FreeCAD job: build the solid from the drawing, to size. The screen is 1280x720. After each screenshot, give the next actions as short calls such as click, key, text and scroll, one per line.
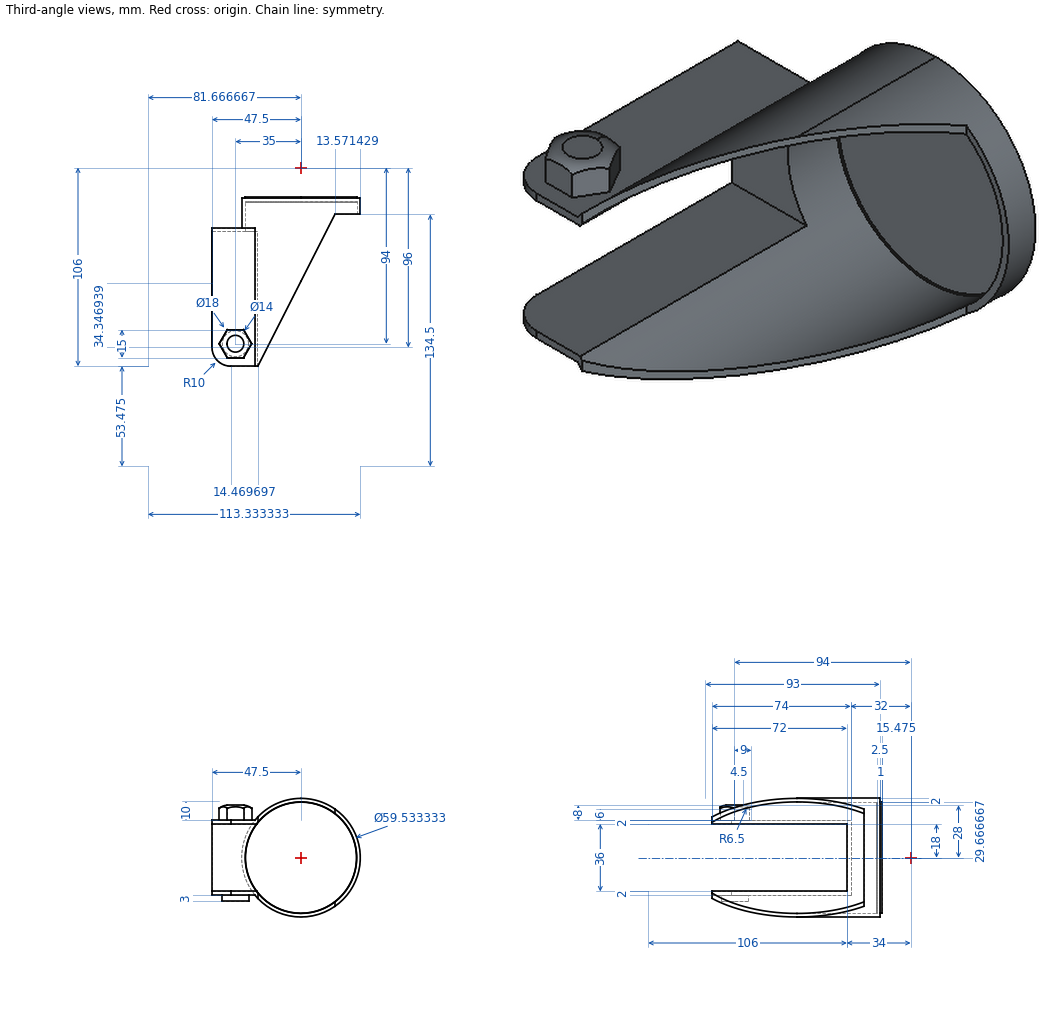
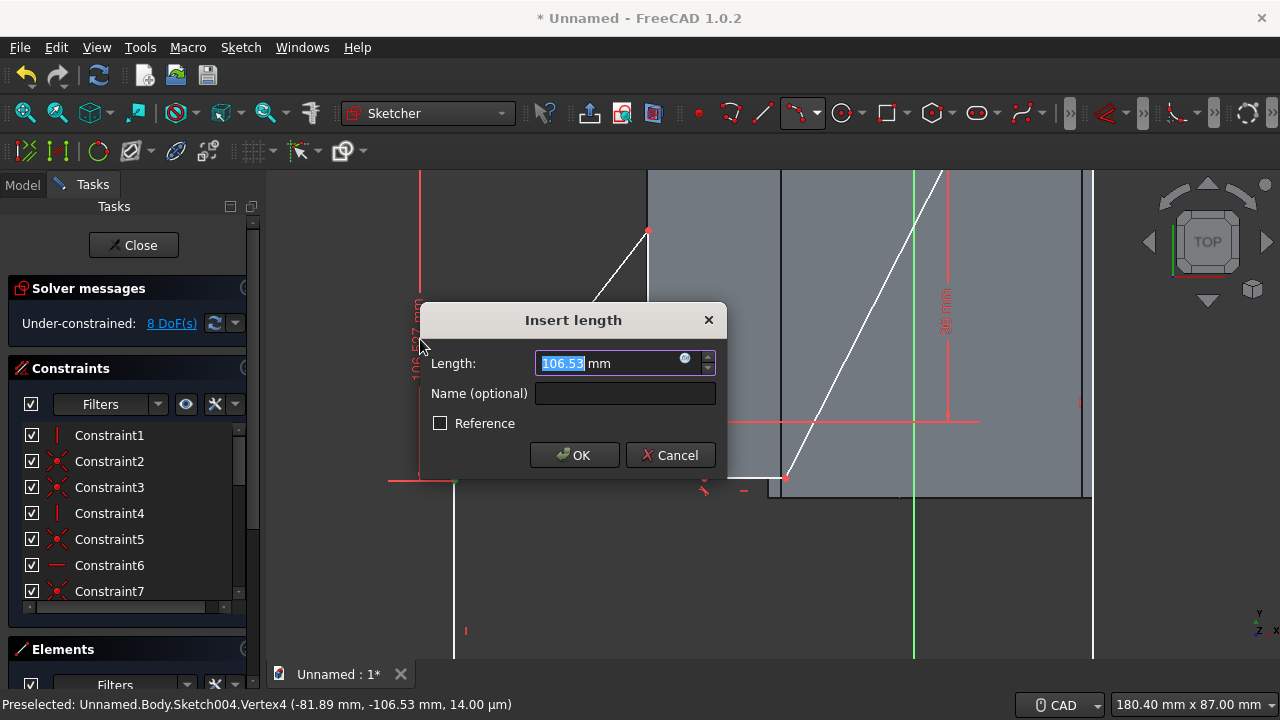
text(106)
key(Return)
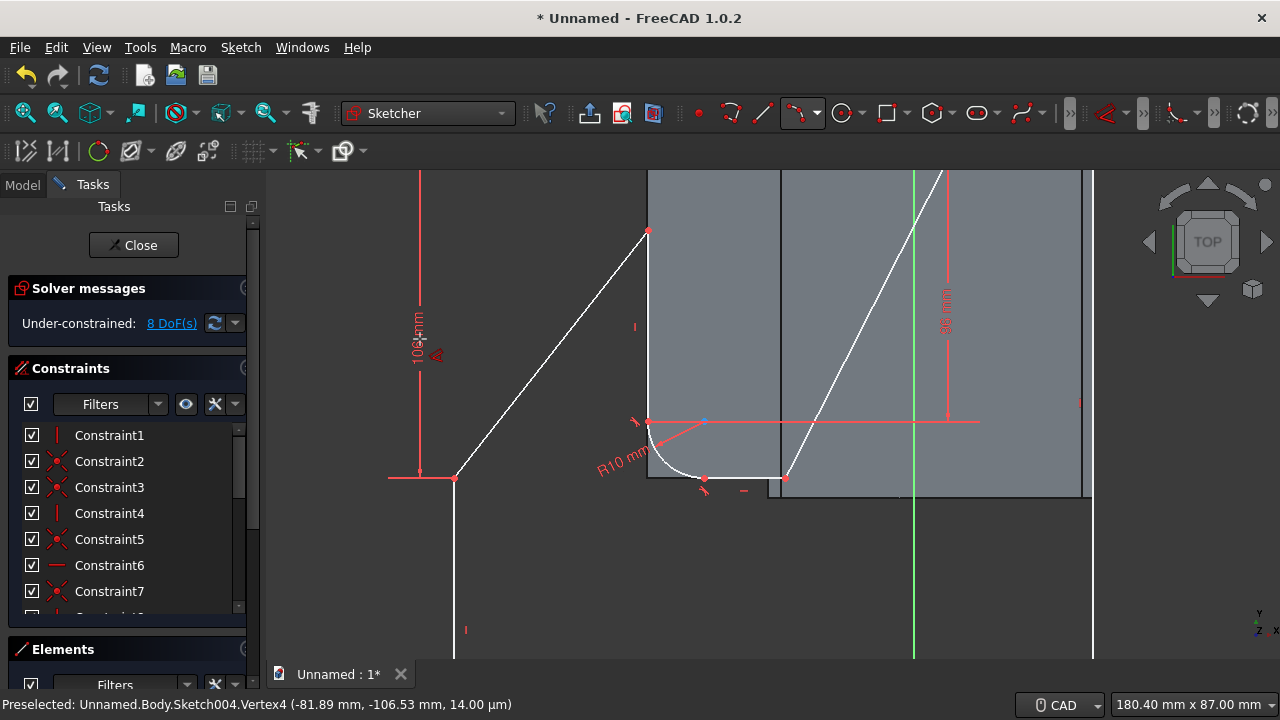
click(1093, 553)
click(1059, 414)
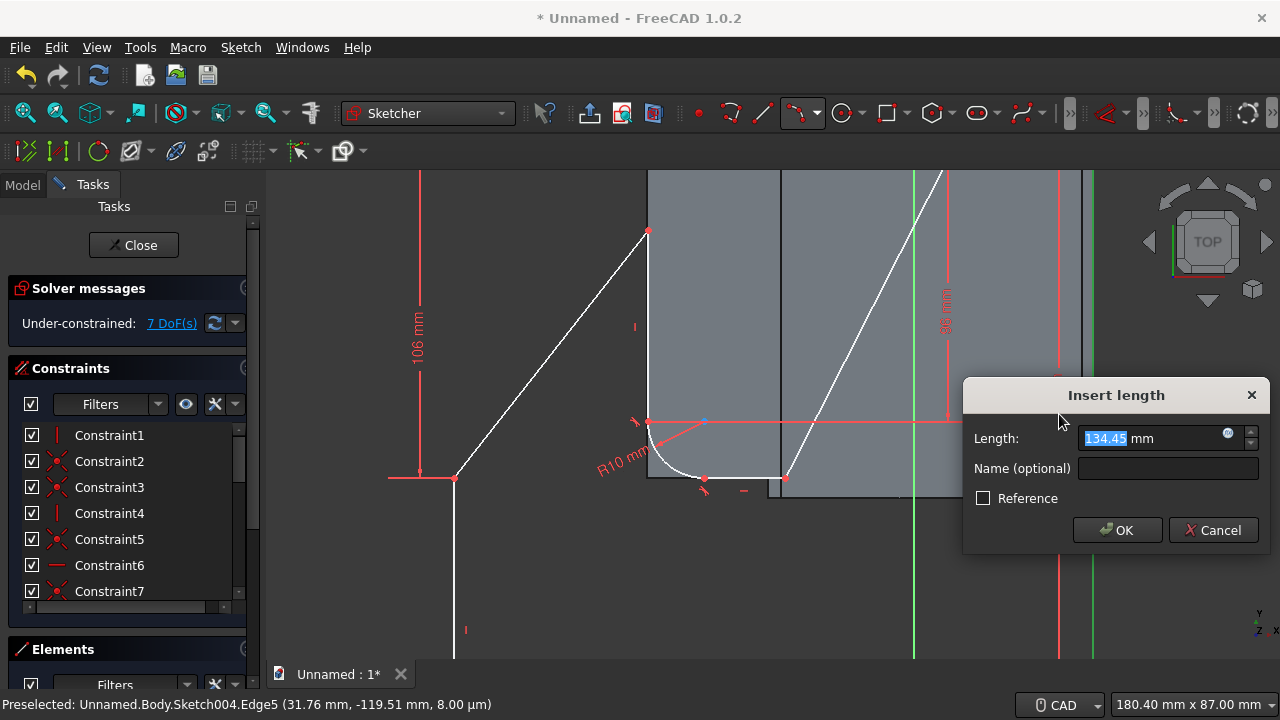
text(134.5)
key(Return)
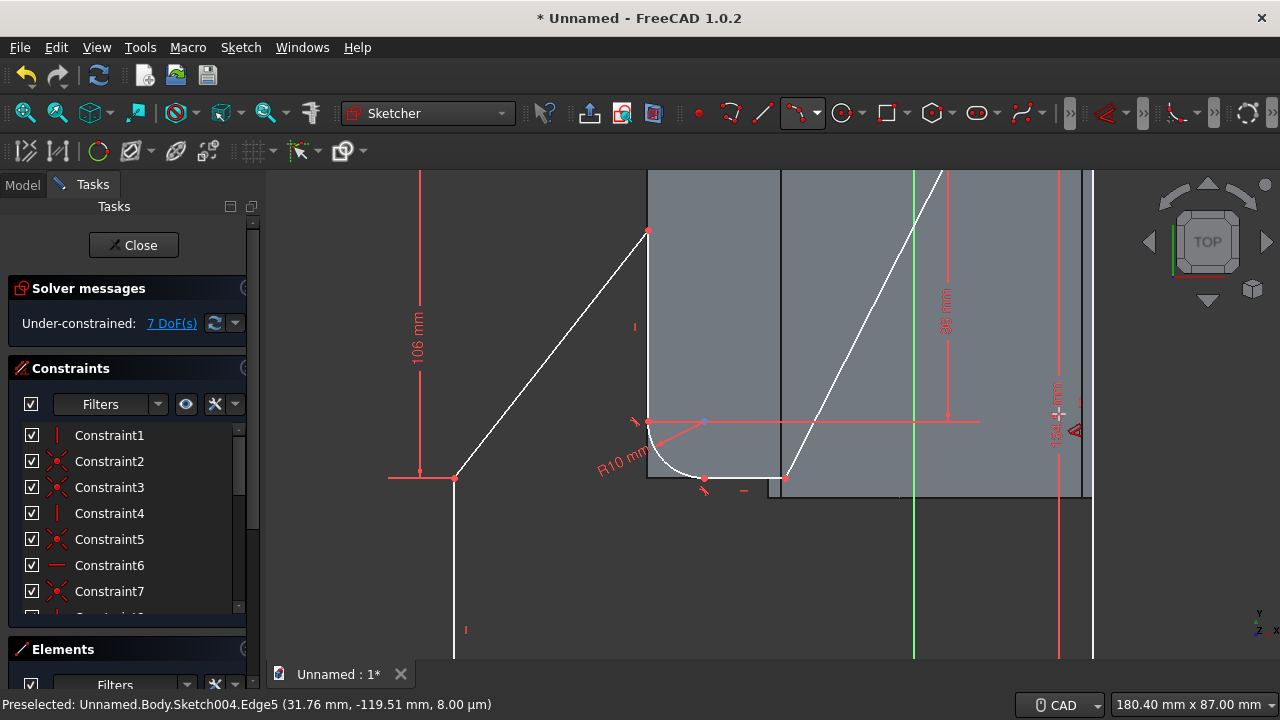
click(648, 422)
click(781, 456)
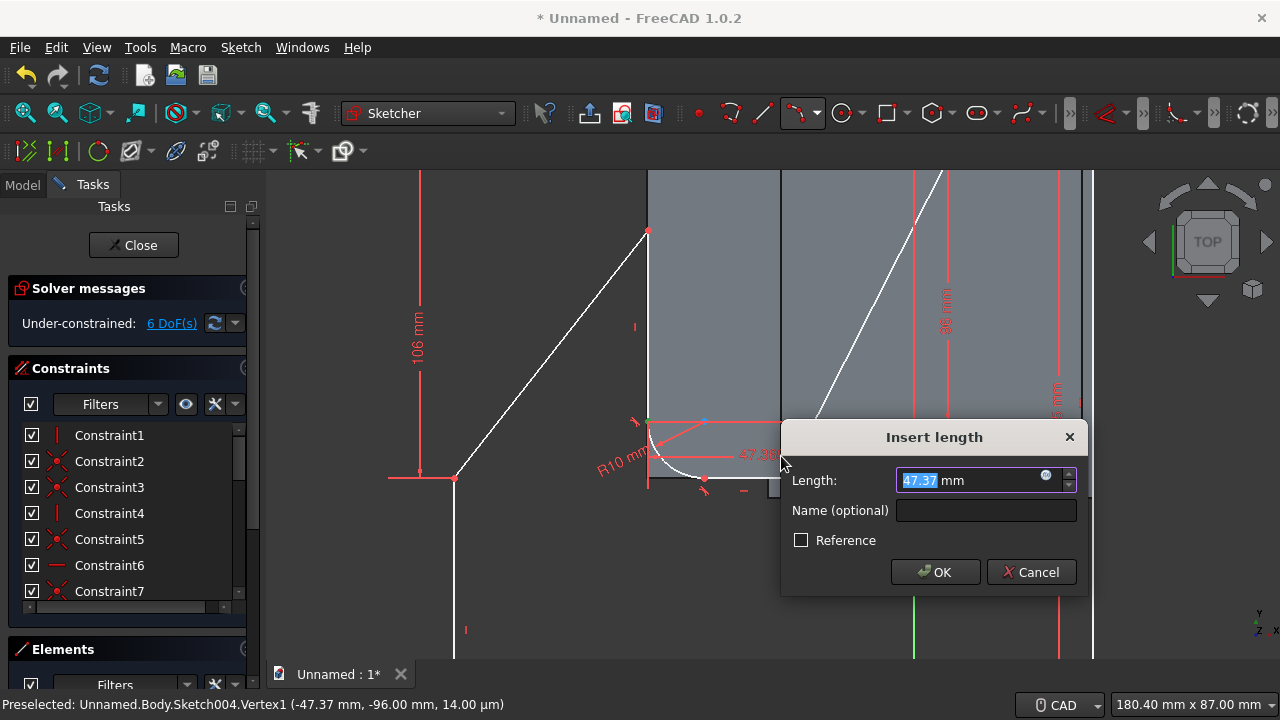
text(47.5)
key(Return)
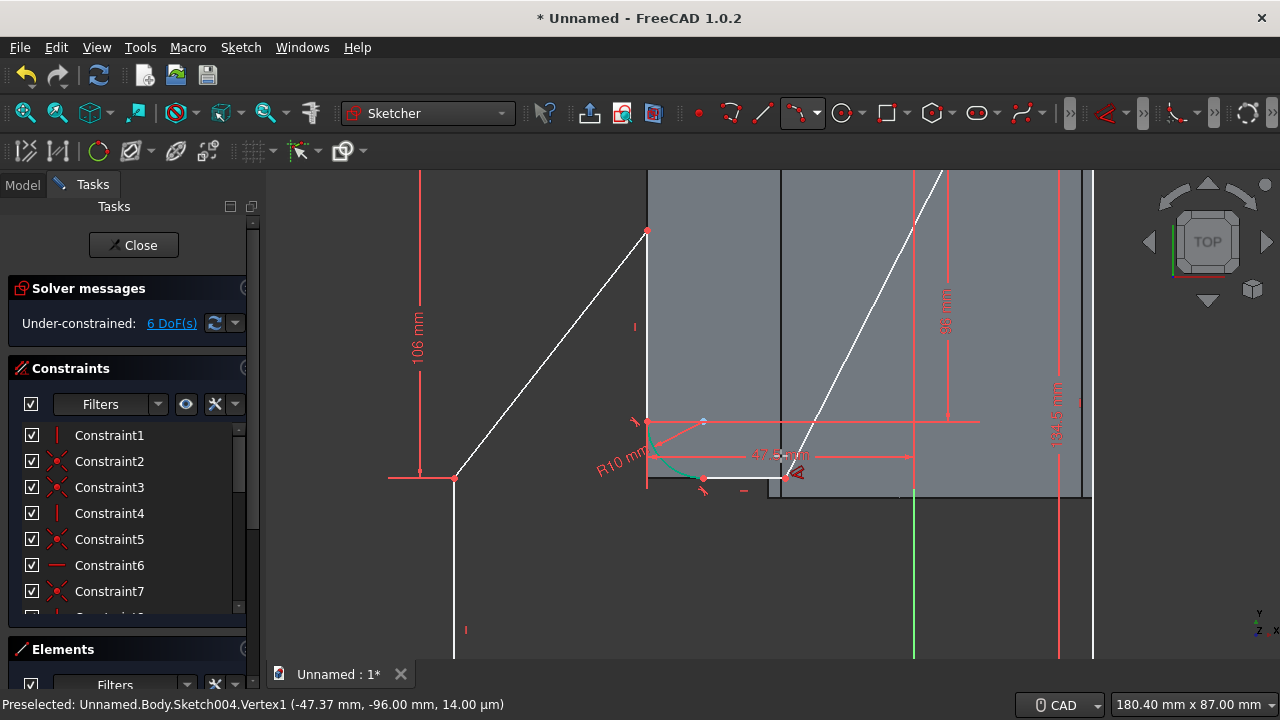
click(454, 569)
click(420, 555)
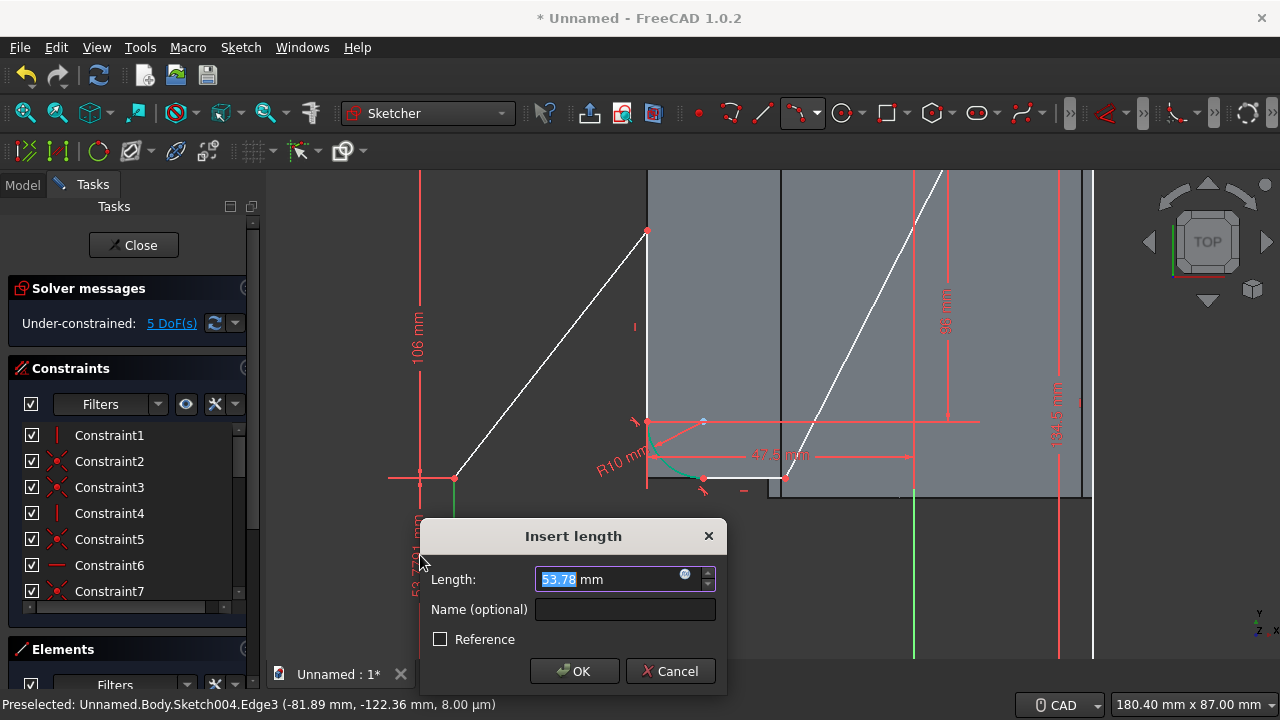
text(53.475)
key(Return)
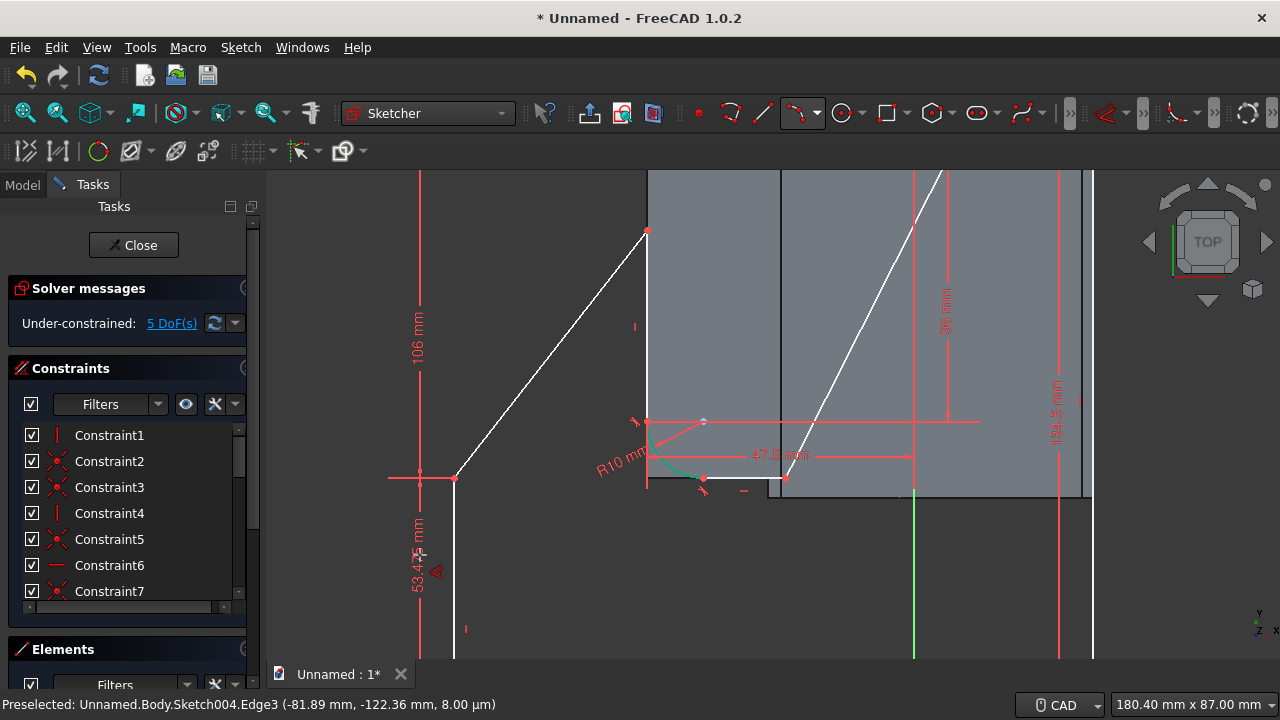
click(647, 365)
click(613, 326)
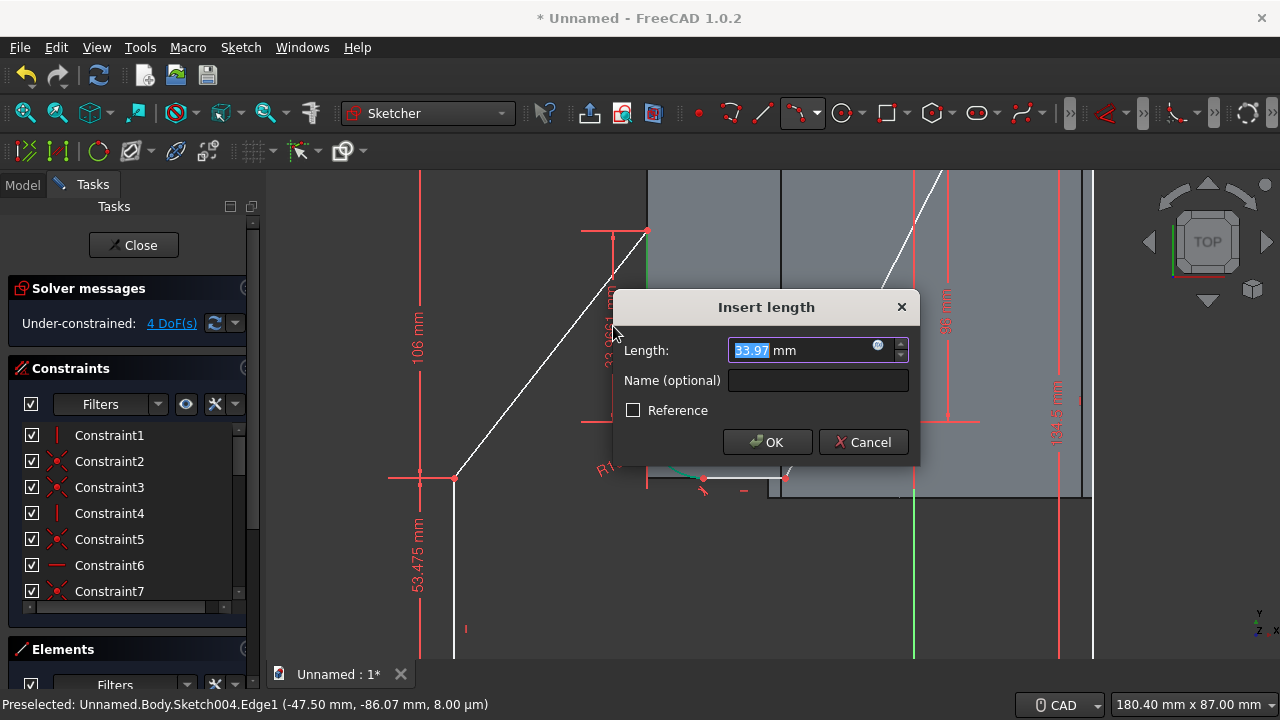
text(34.346939)
key(Return)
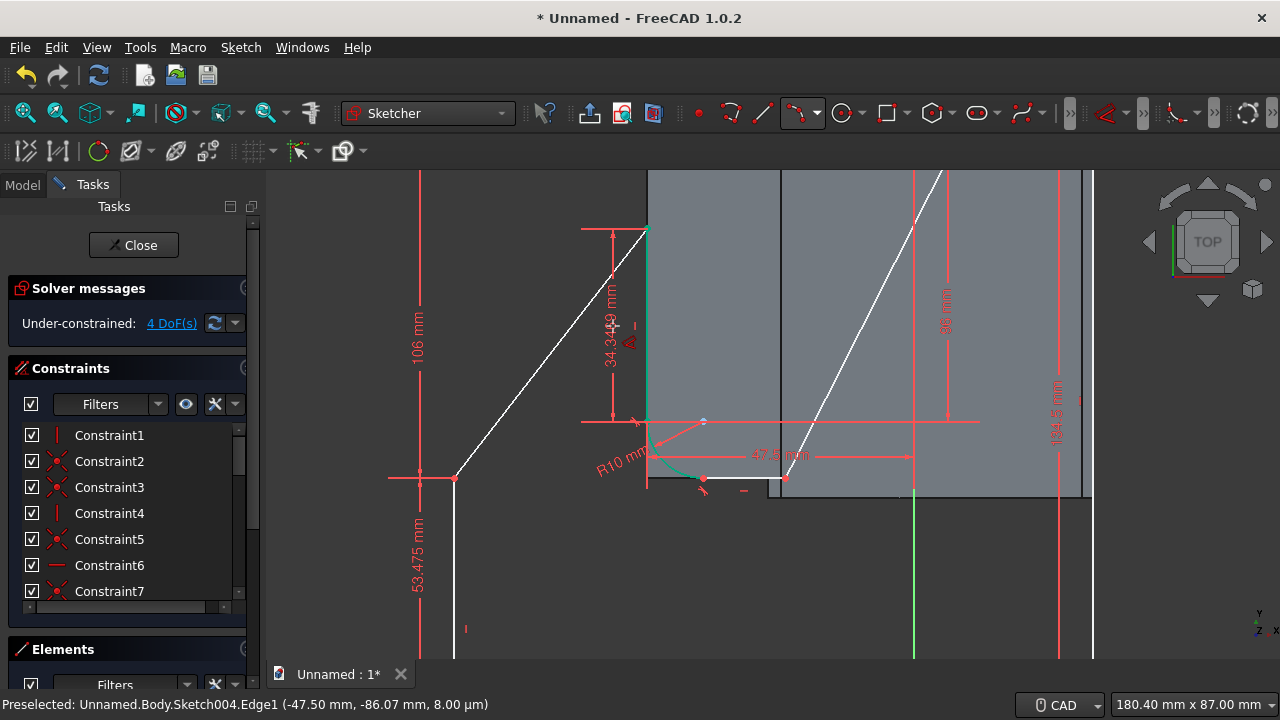
scroll(664, 463, down, 5)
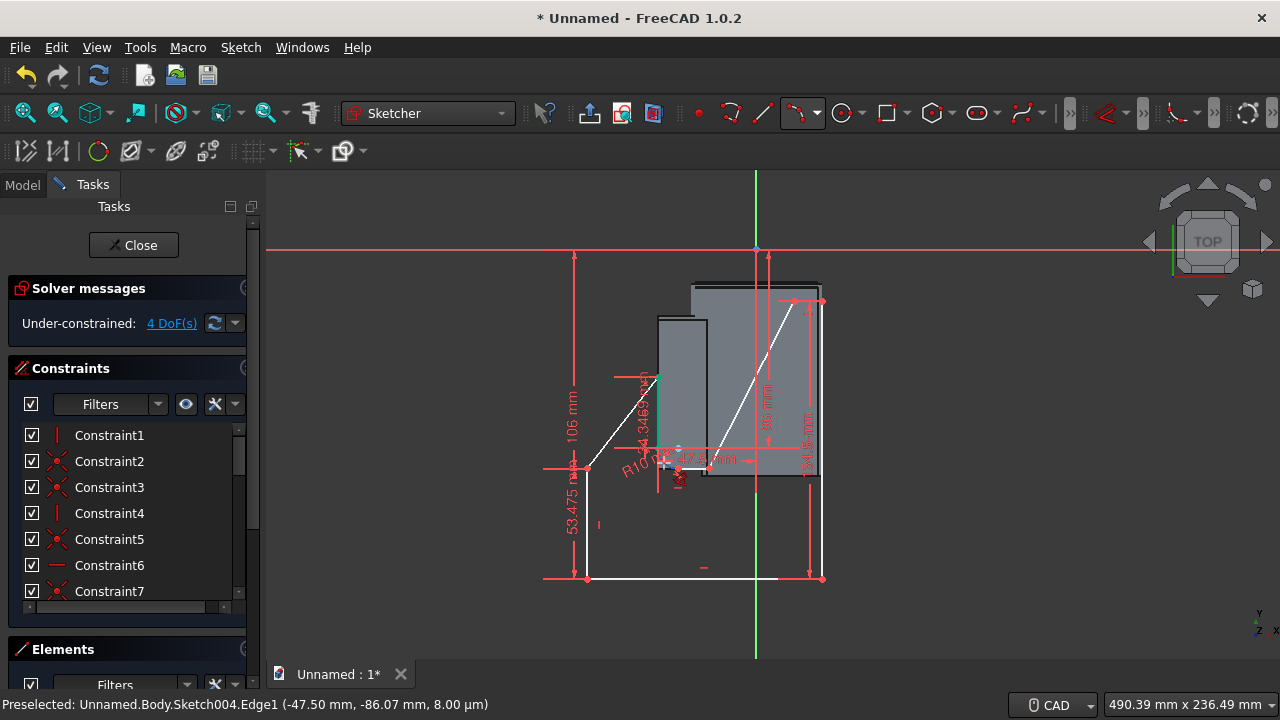
scroll(814, 301, up, 3)